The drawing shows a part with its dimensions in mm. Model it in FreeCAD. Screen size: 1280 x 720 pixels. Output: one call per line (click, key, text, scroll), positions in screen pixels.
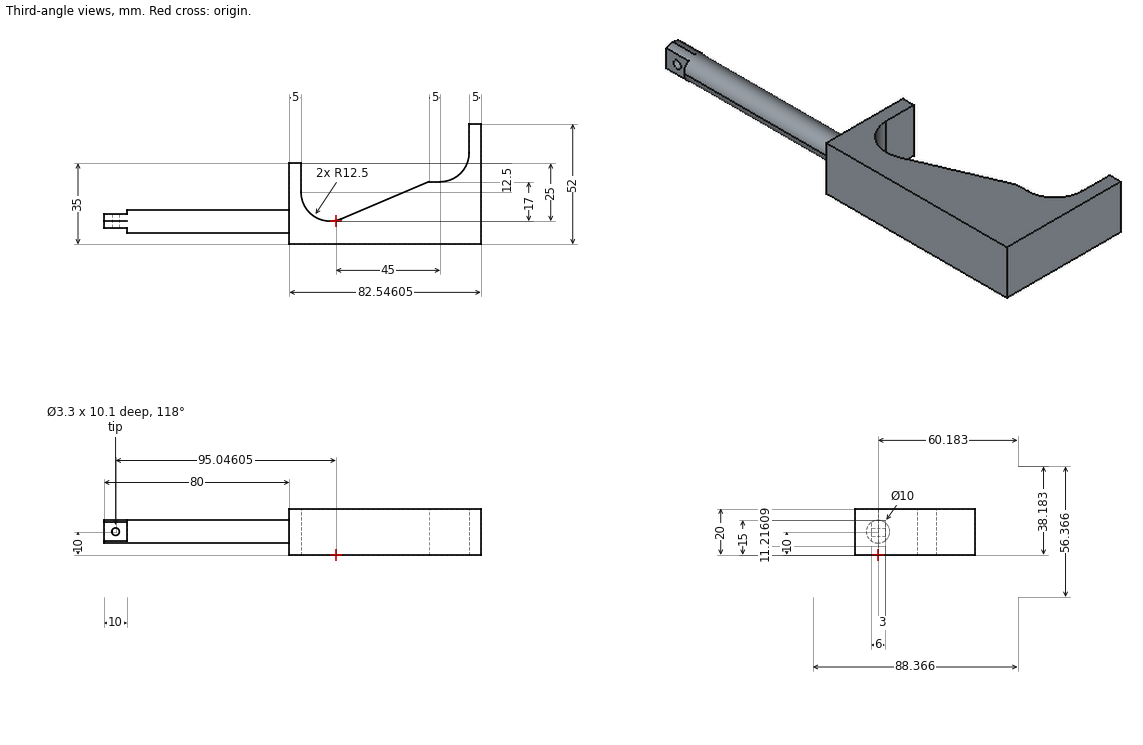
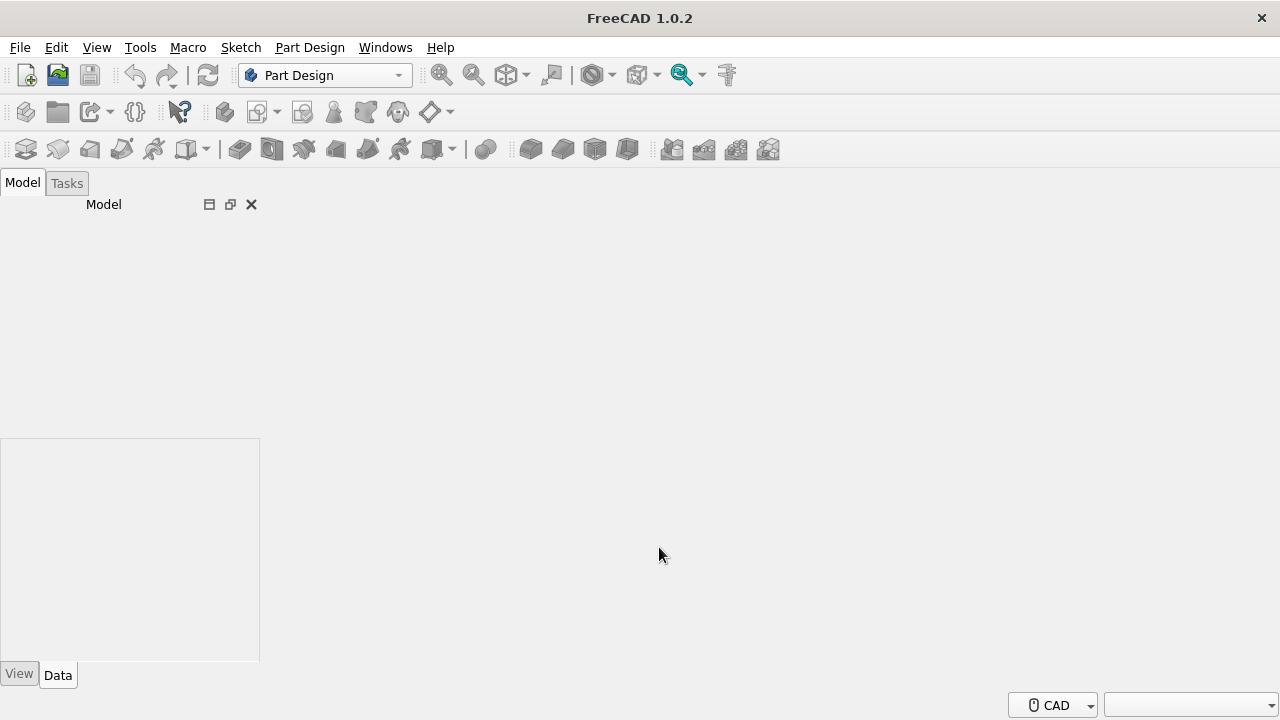
click(26, 76)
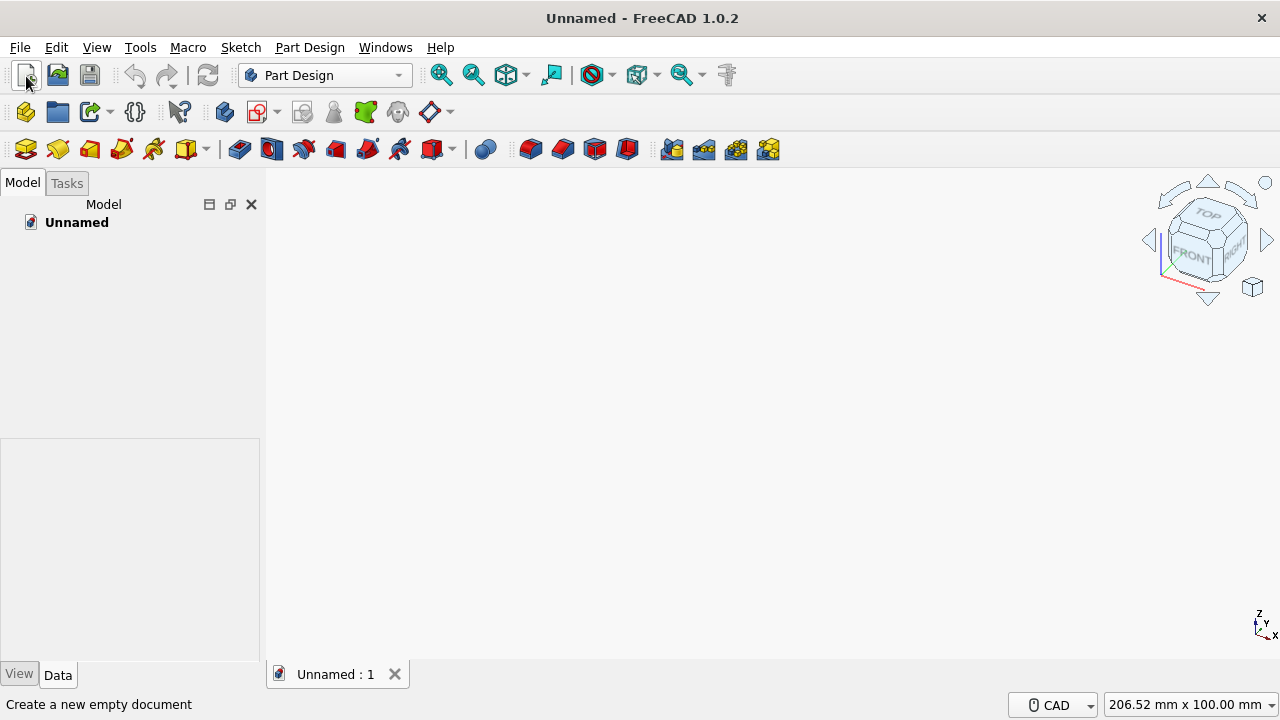
click(258, 112)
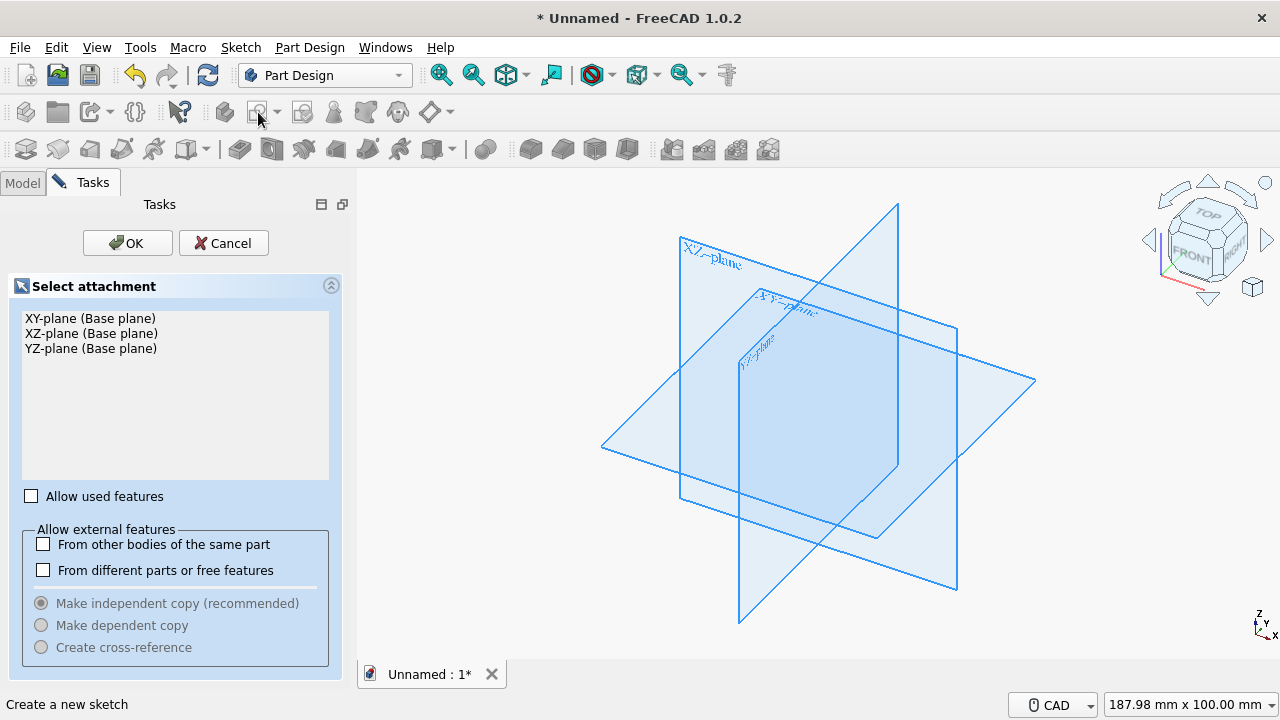
click(82, 318)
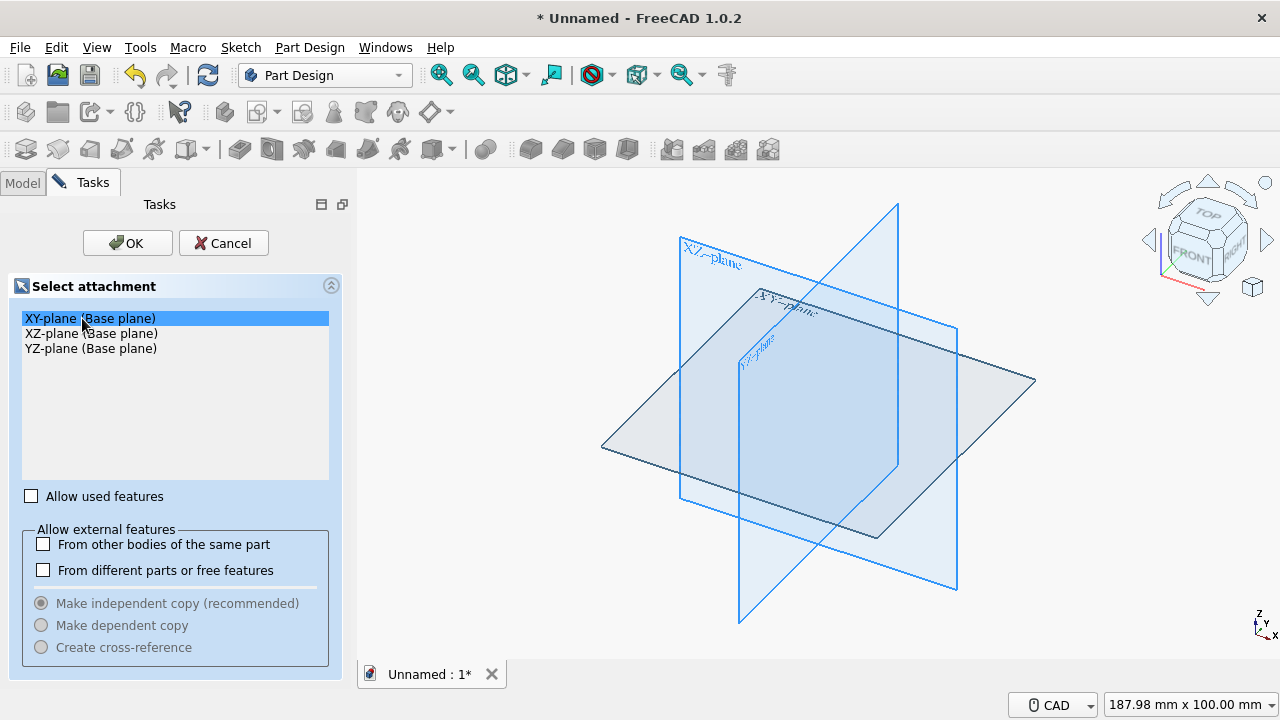
click(128, 243)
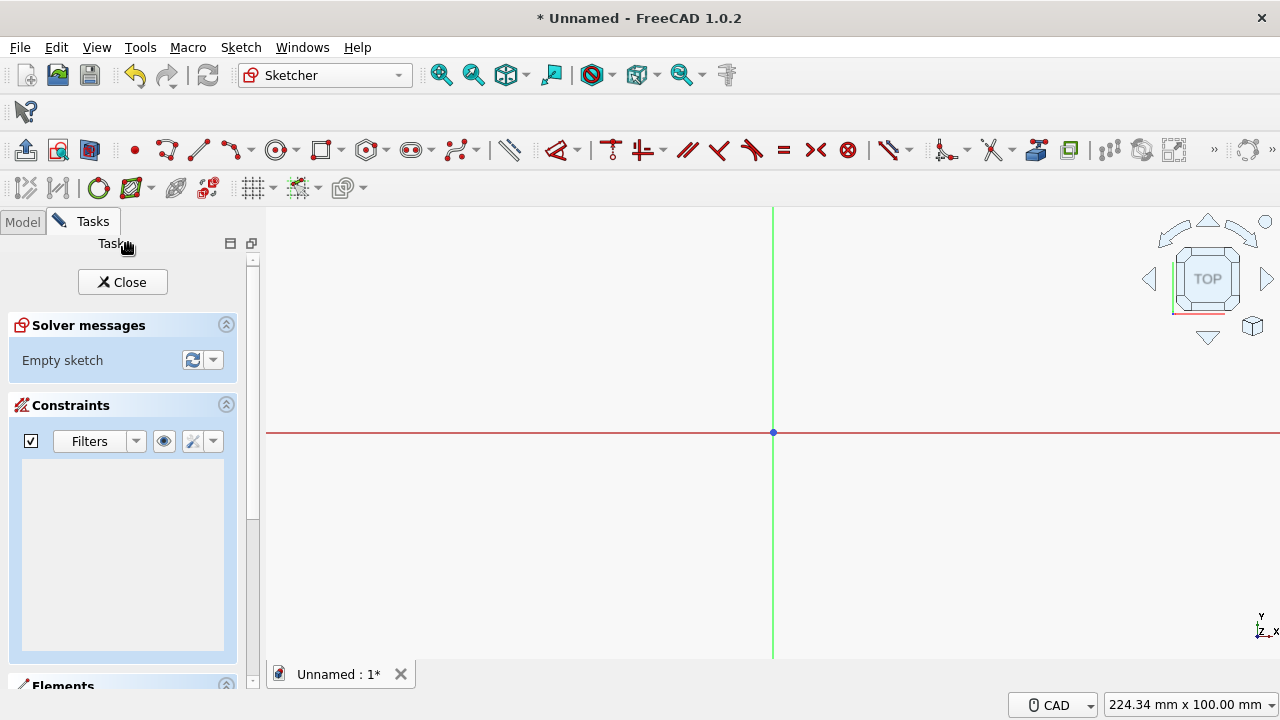
scroll(294, 631, down, 1)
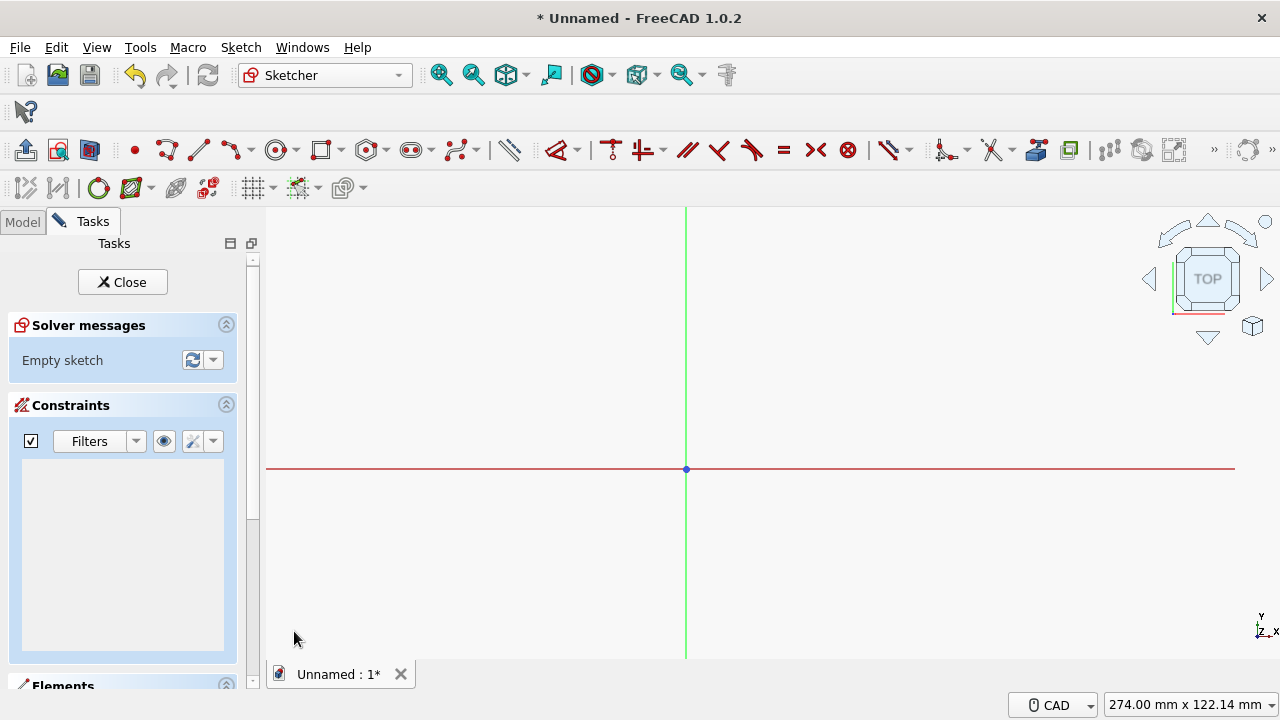
scroll(887, 363, up, 2)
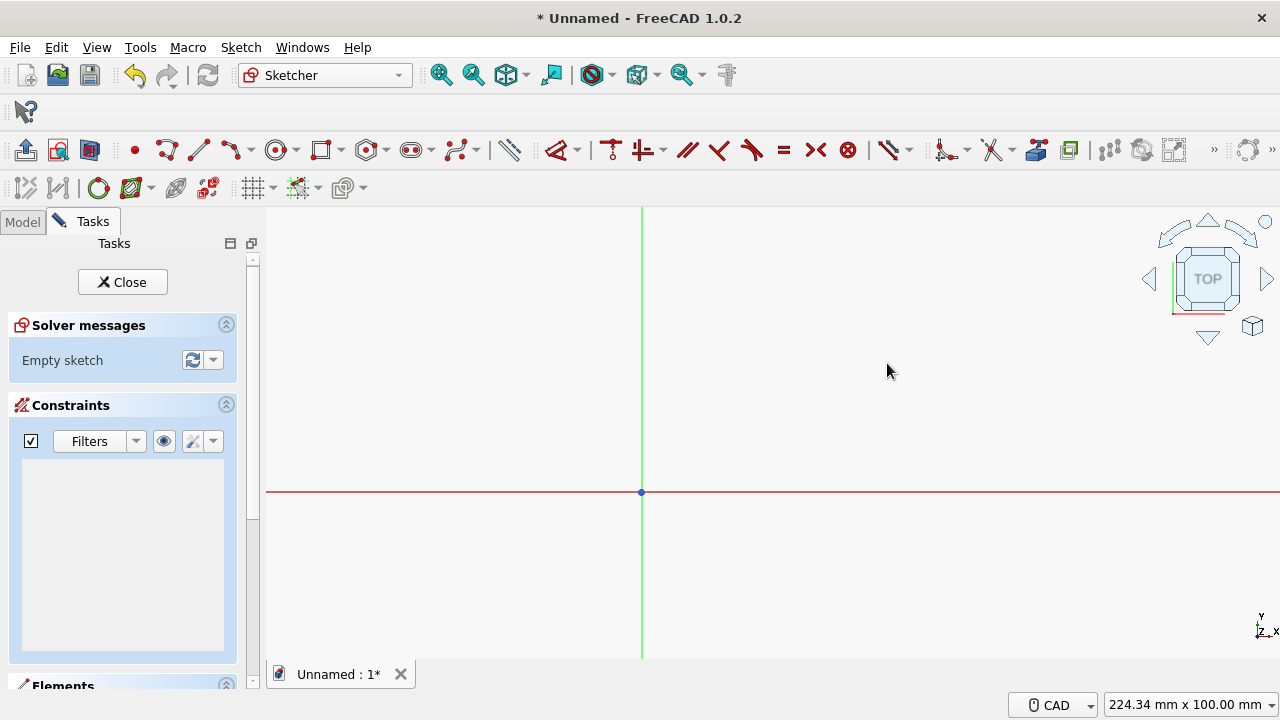
click(168, 150)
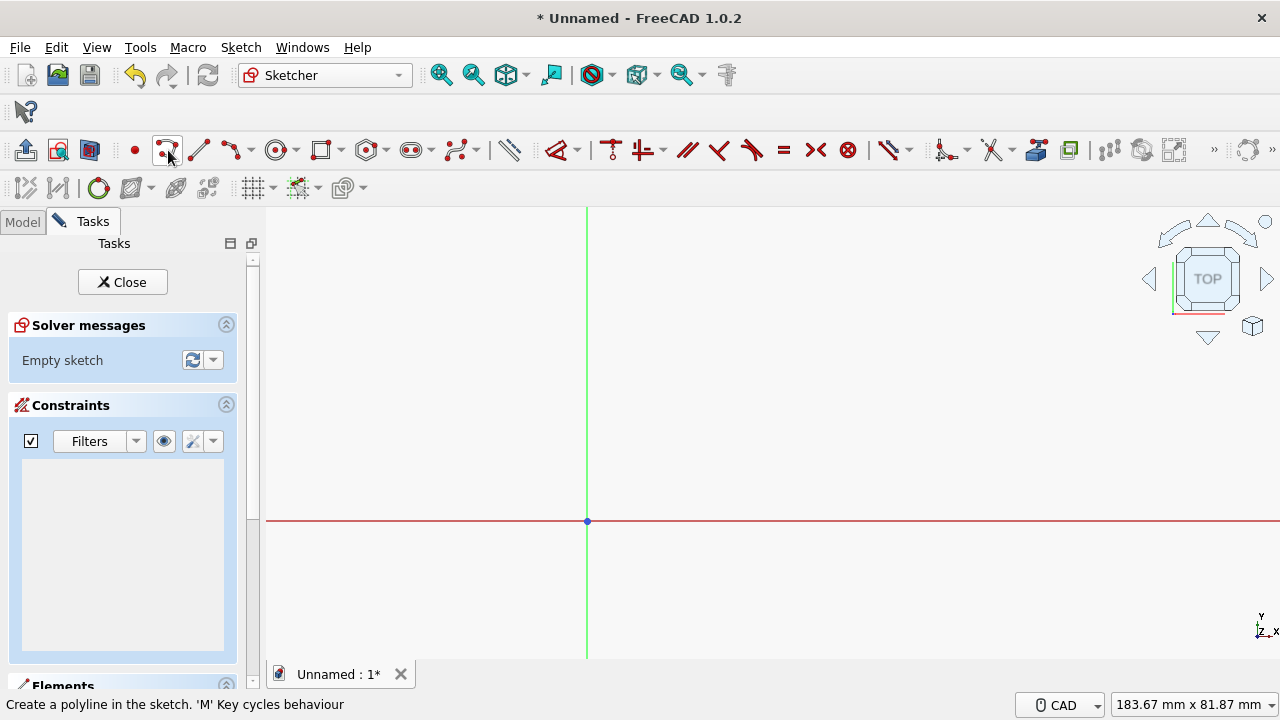
click(504, 452)
click(504, 383)
click(476, 383)
click(476, 576)
click(932, 576)
click(932, 289)
click(905, 289)
click(905, 358)
right_click(905, 358)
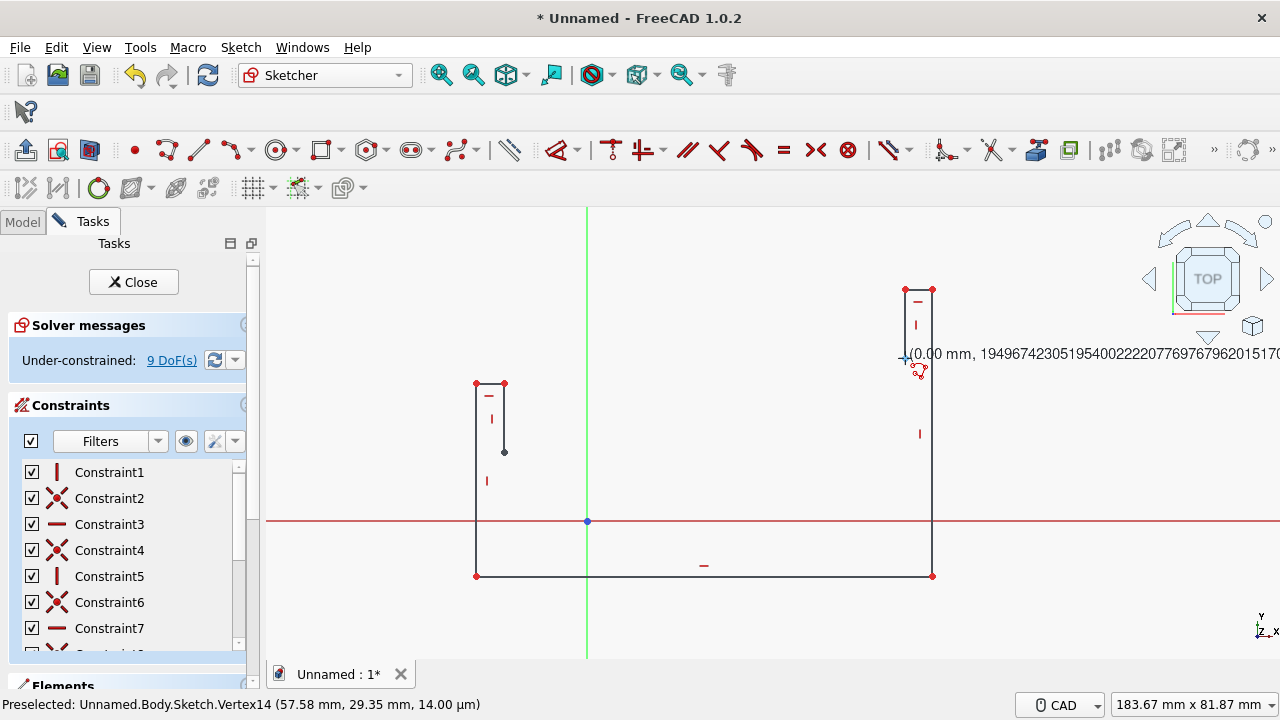
click(836, 427)
click(808, 427)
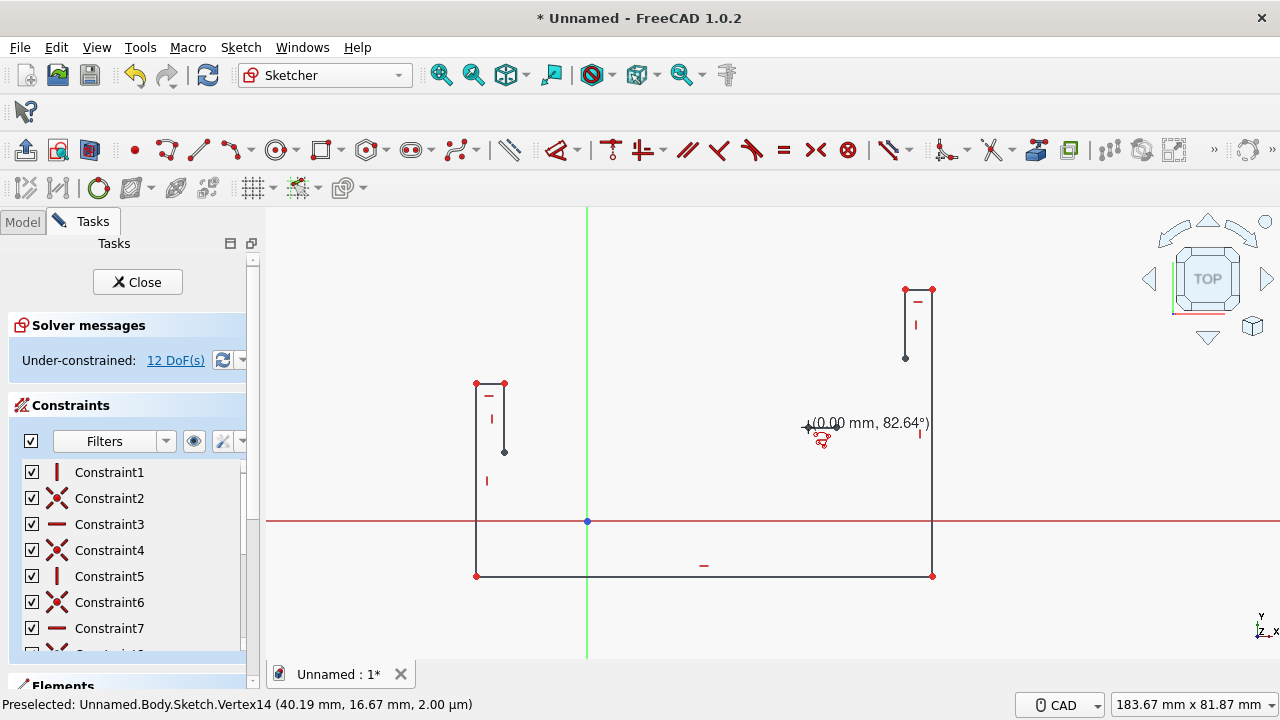
scroll(600, 516, up, 6)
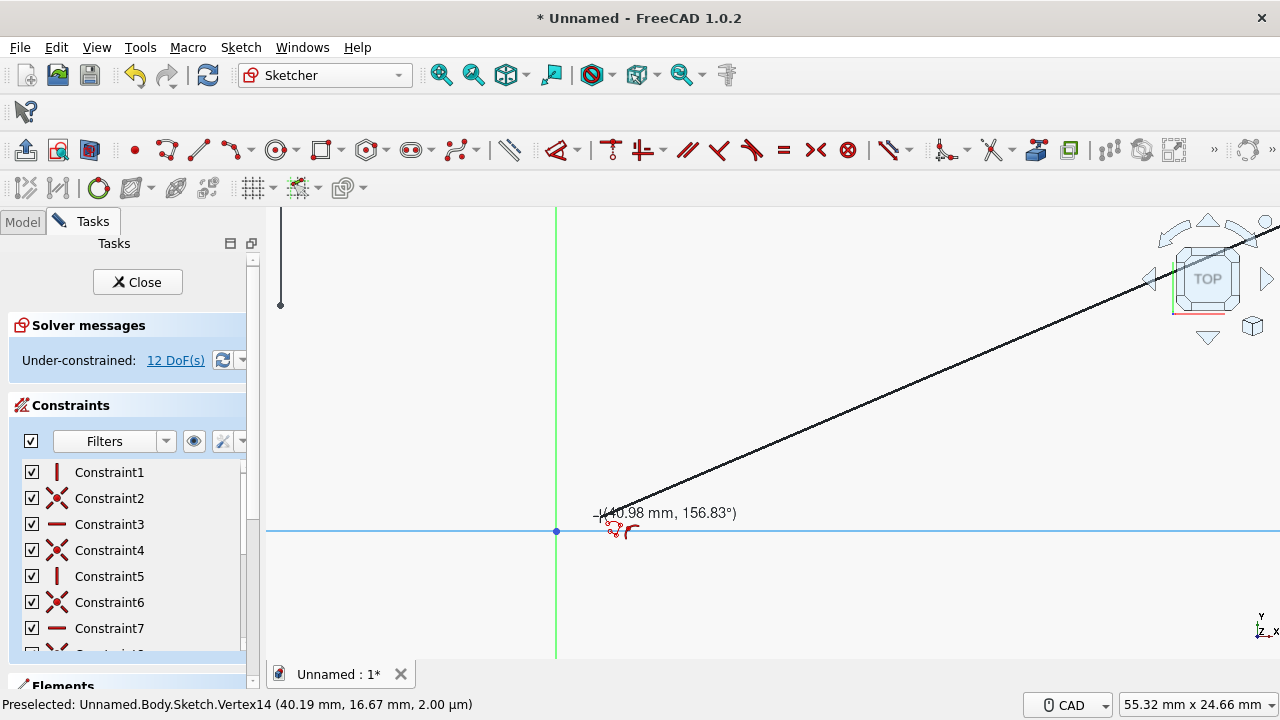
click(599, 513)
right_click(599, 513)